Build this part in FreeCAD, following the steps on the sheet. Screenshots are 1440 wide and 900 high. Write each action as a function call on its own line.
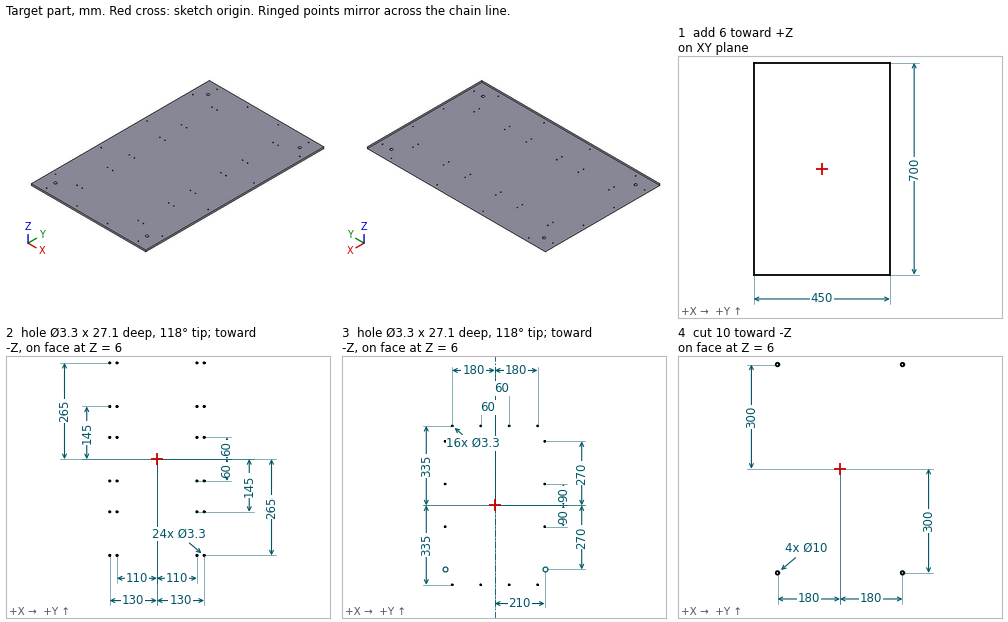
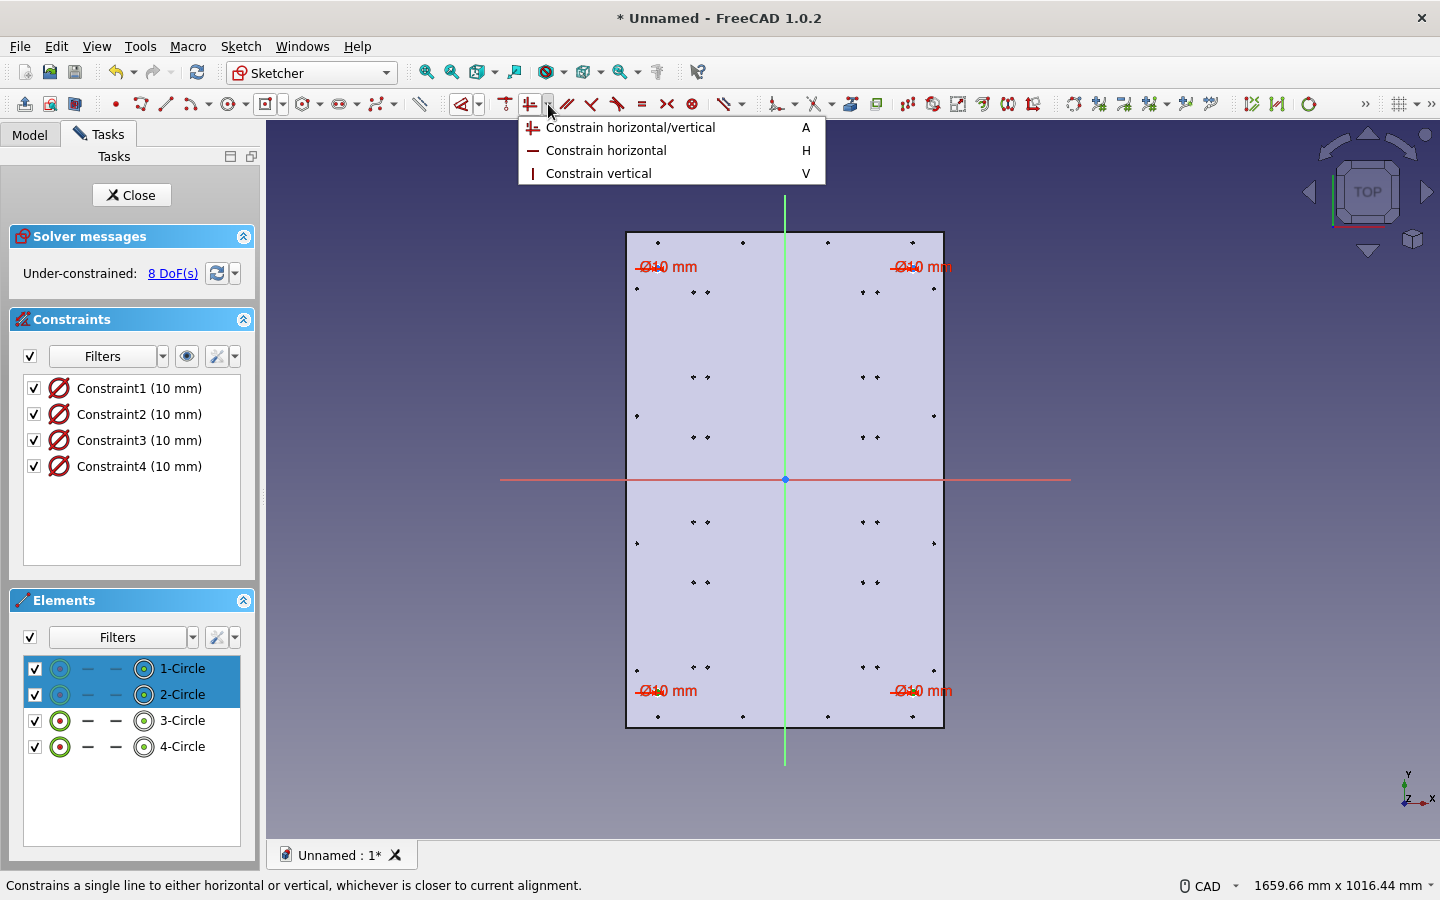
click(672, 150)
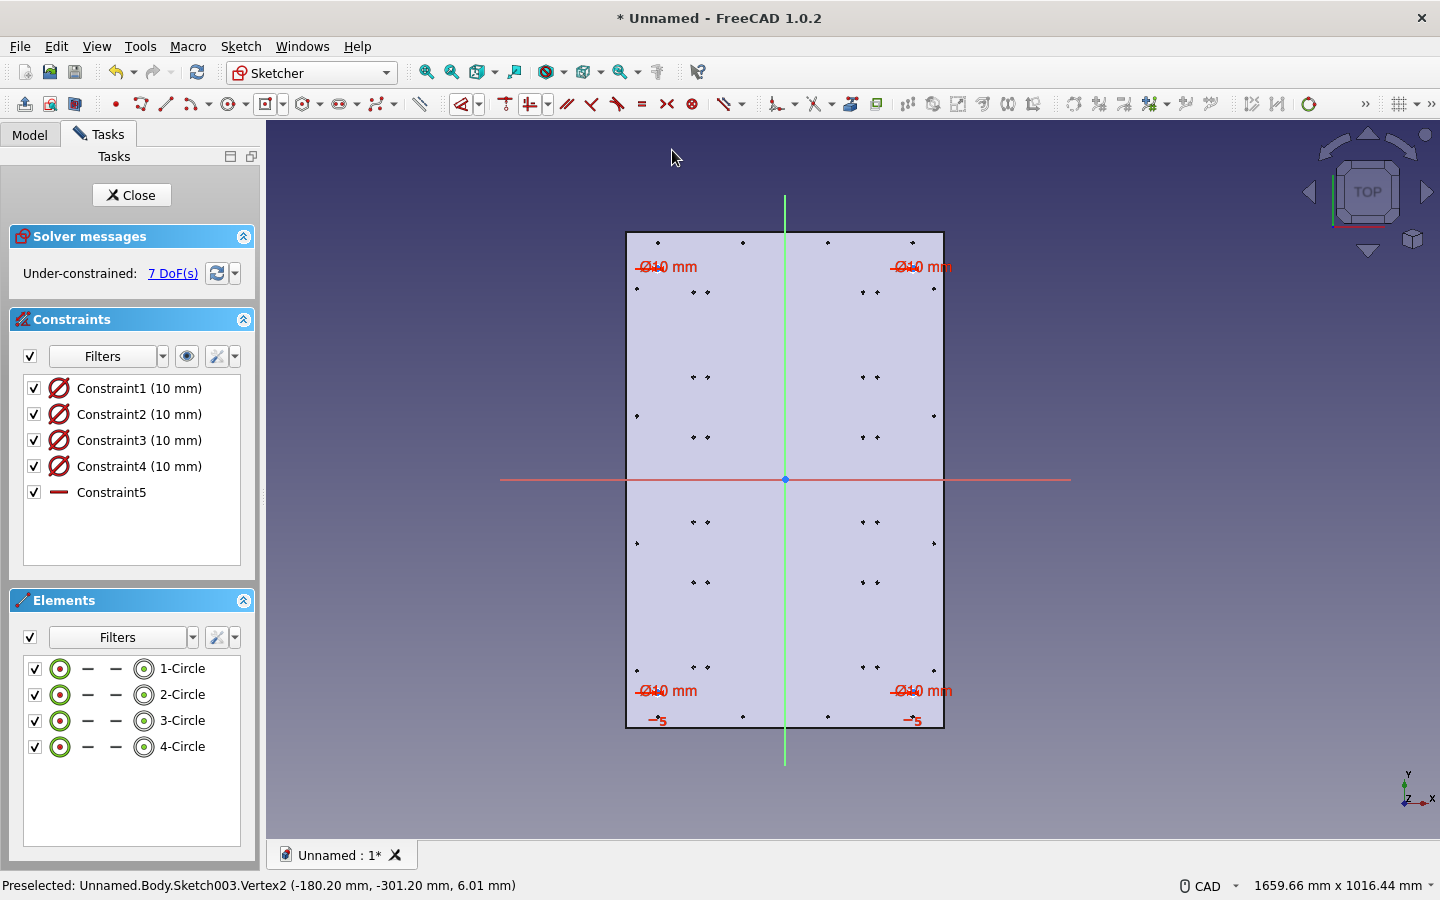
click(658, 693)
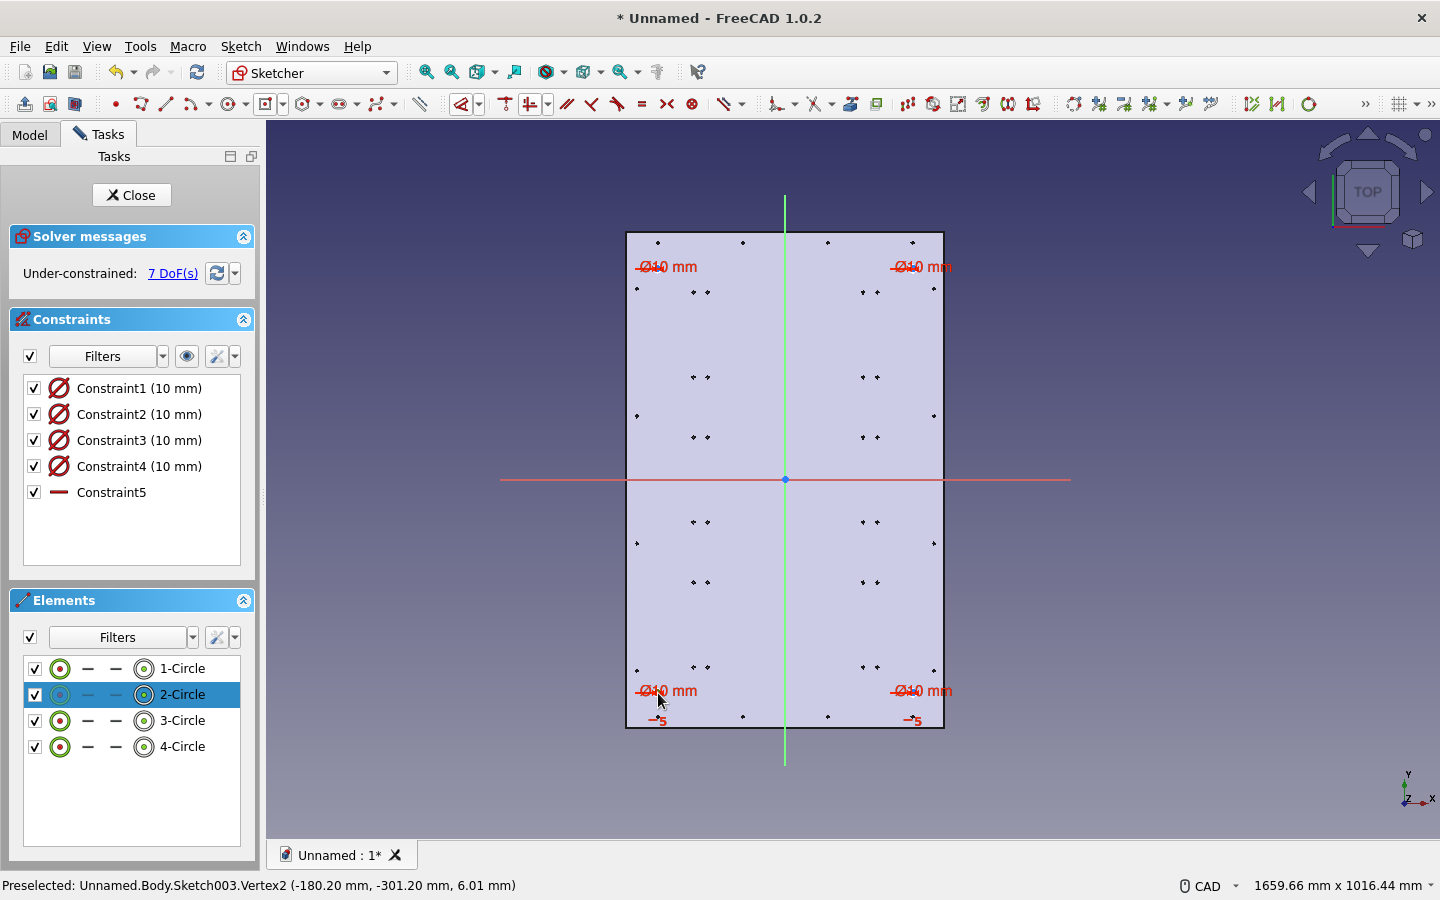
click(658, 269)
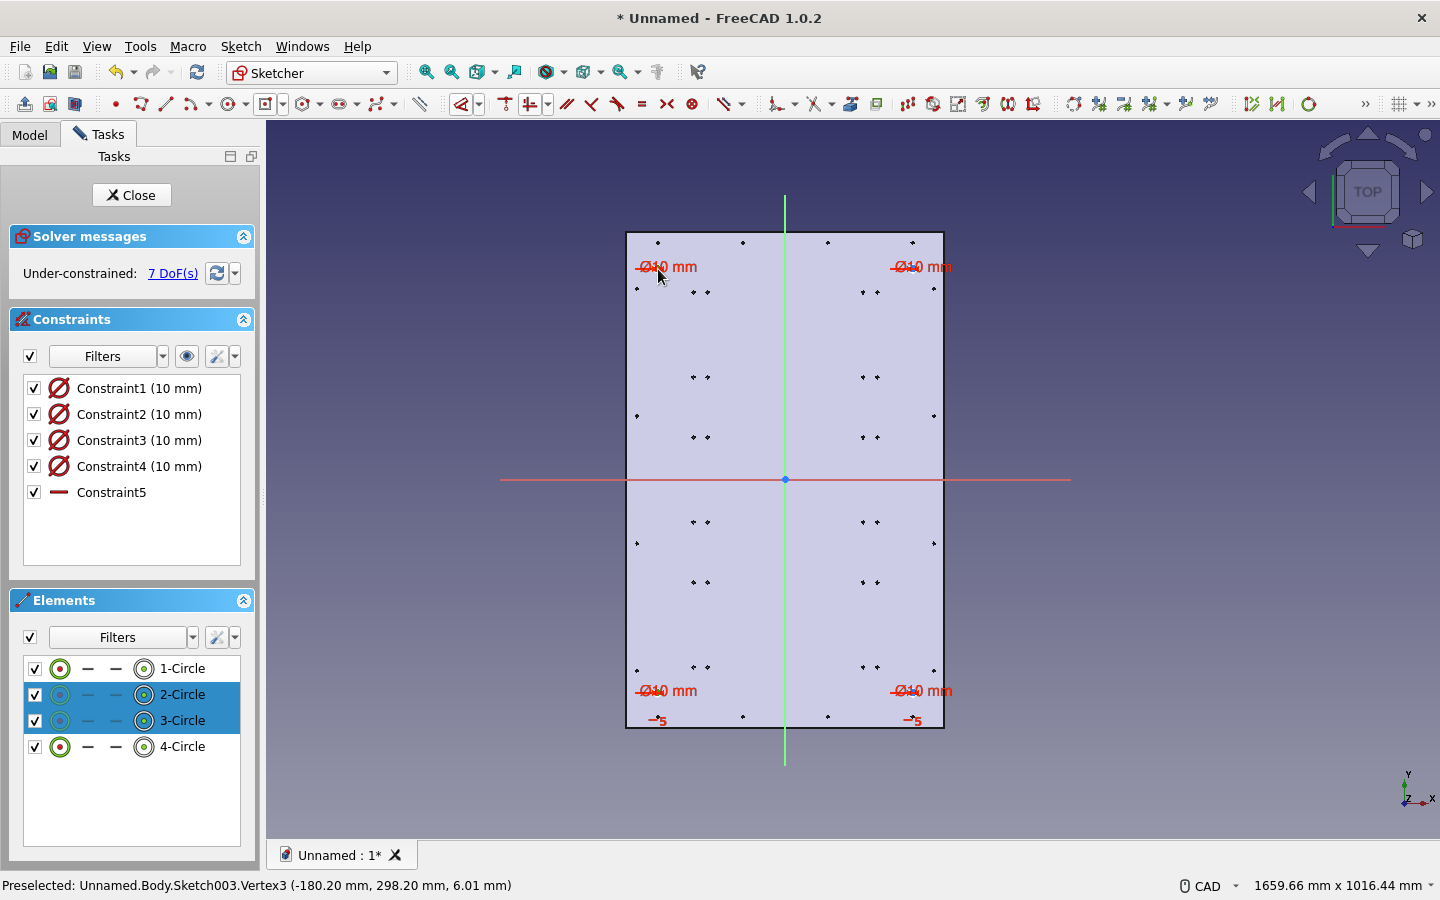
click(548, 104)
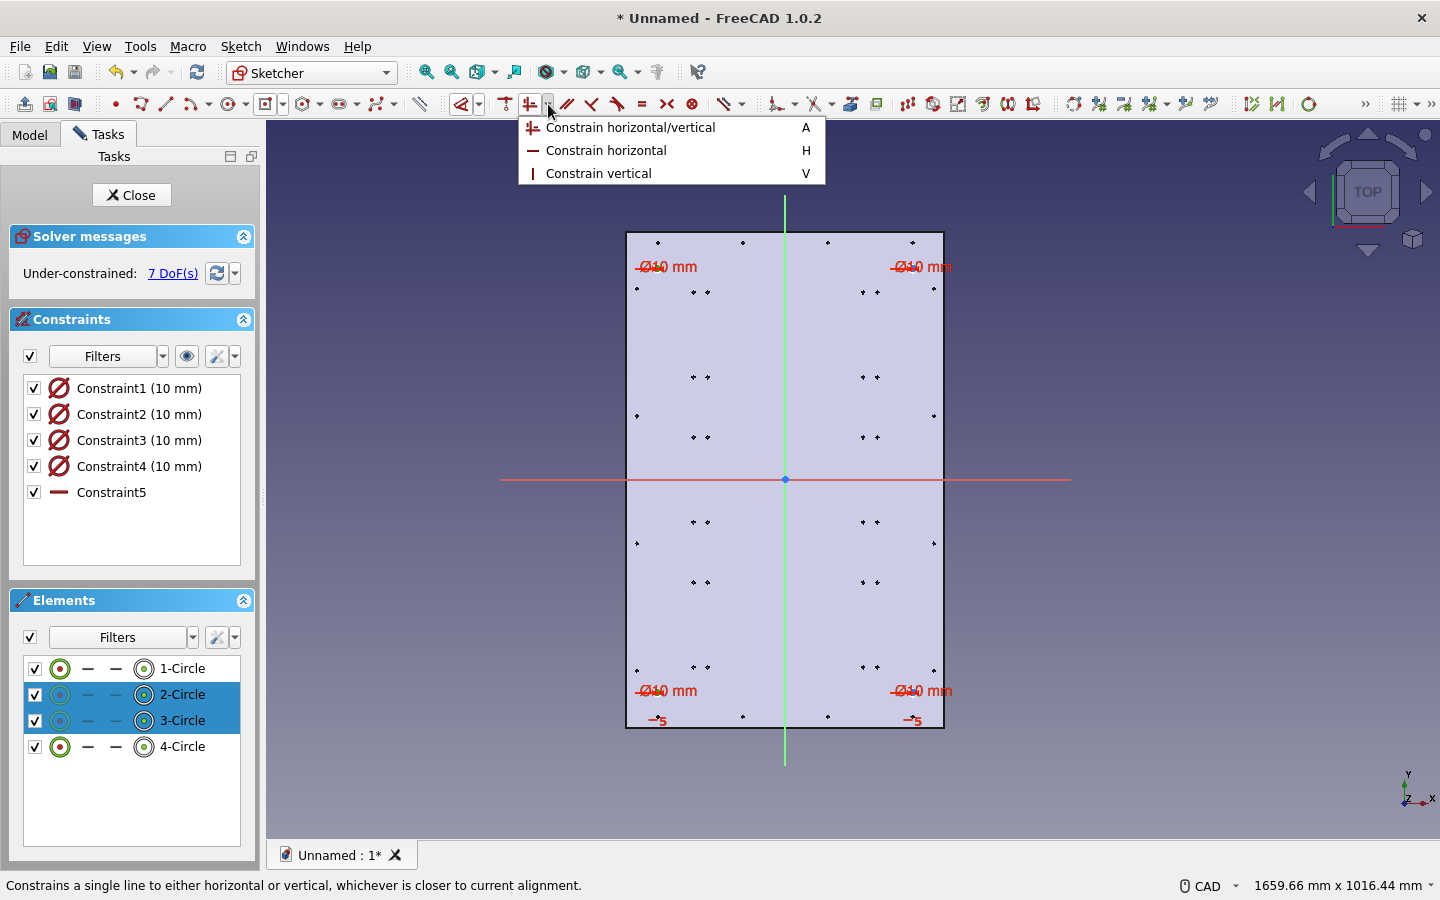
click(672, 174)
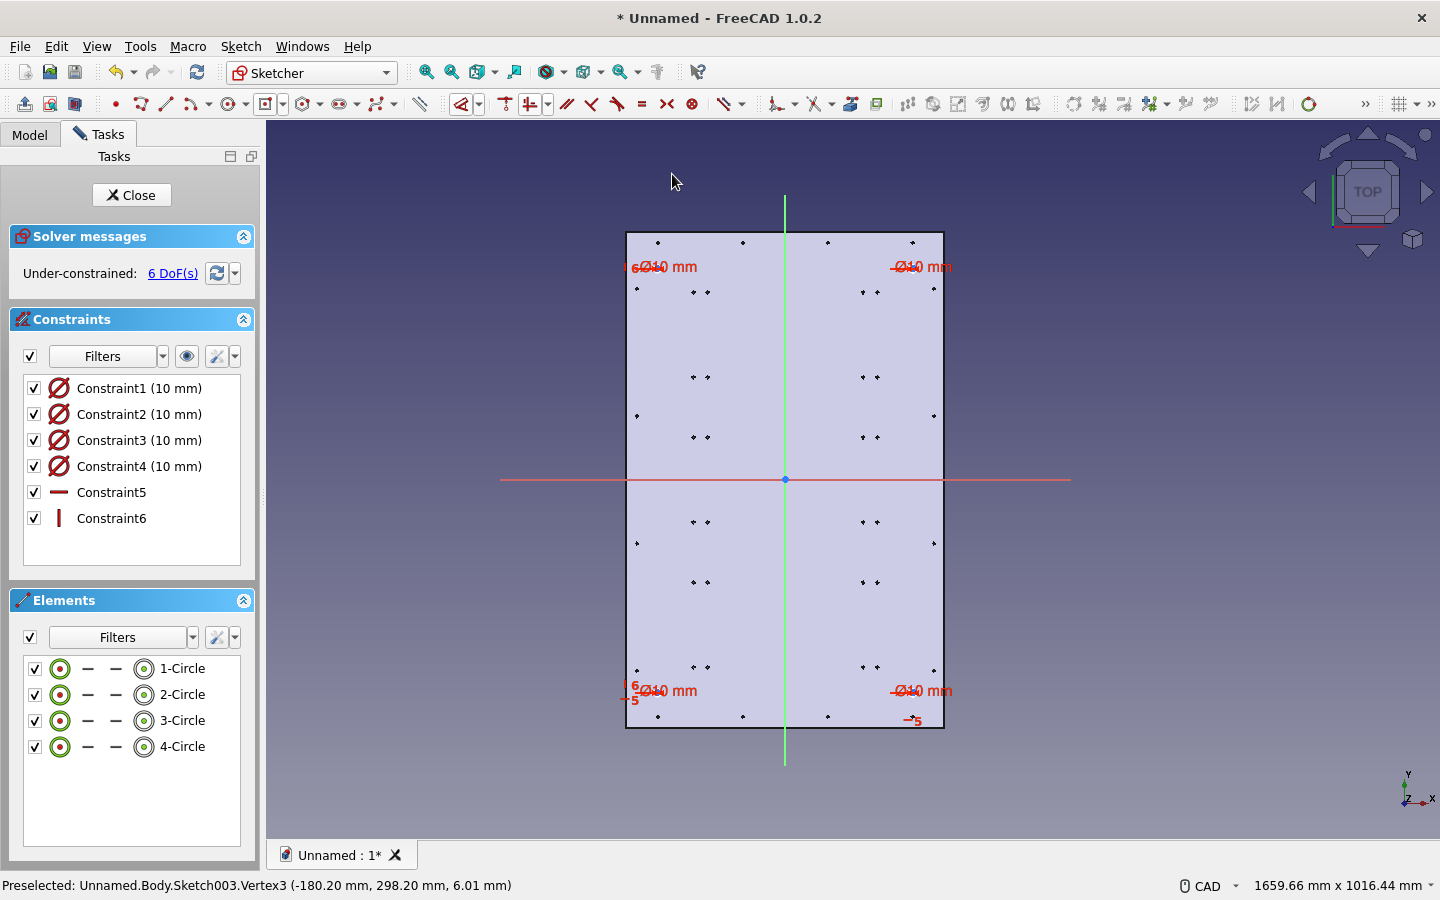
click(913, 693)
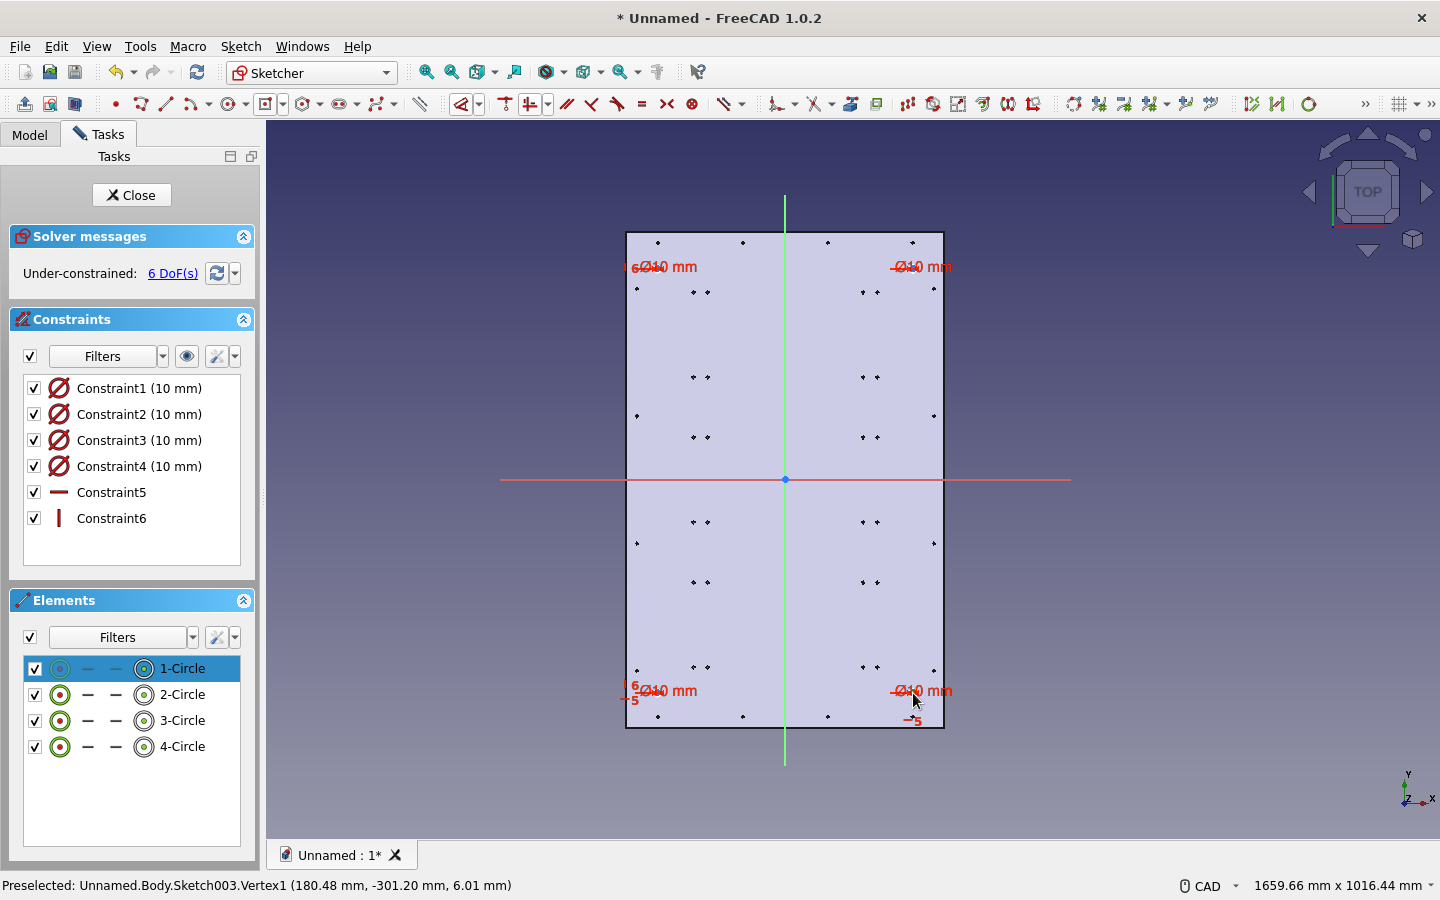
click(913, 269)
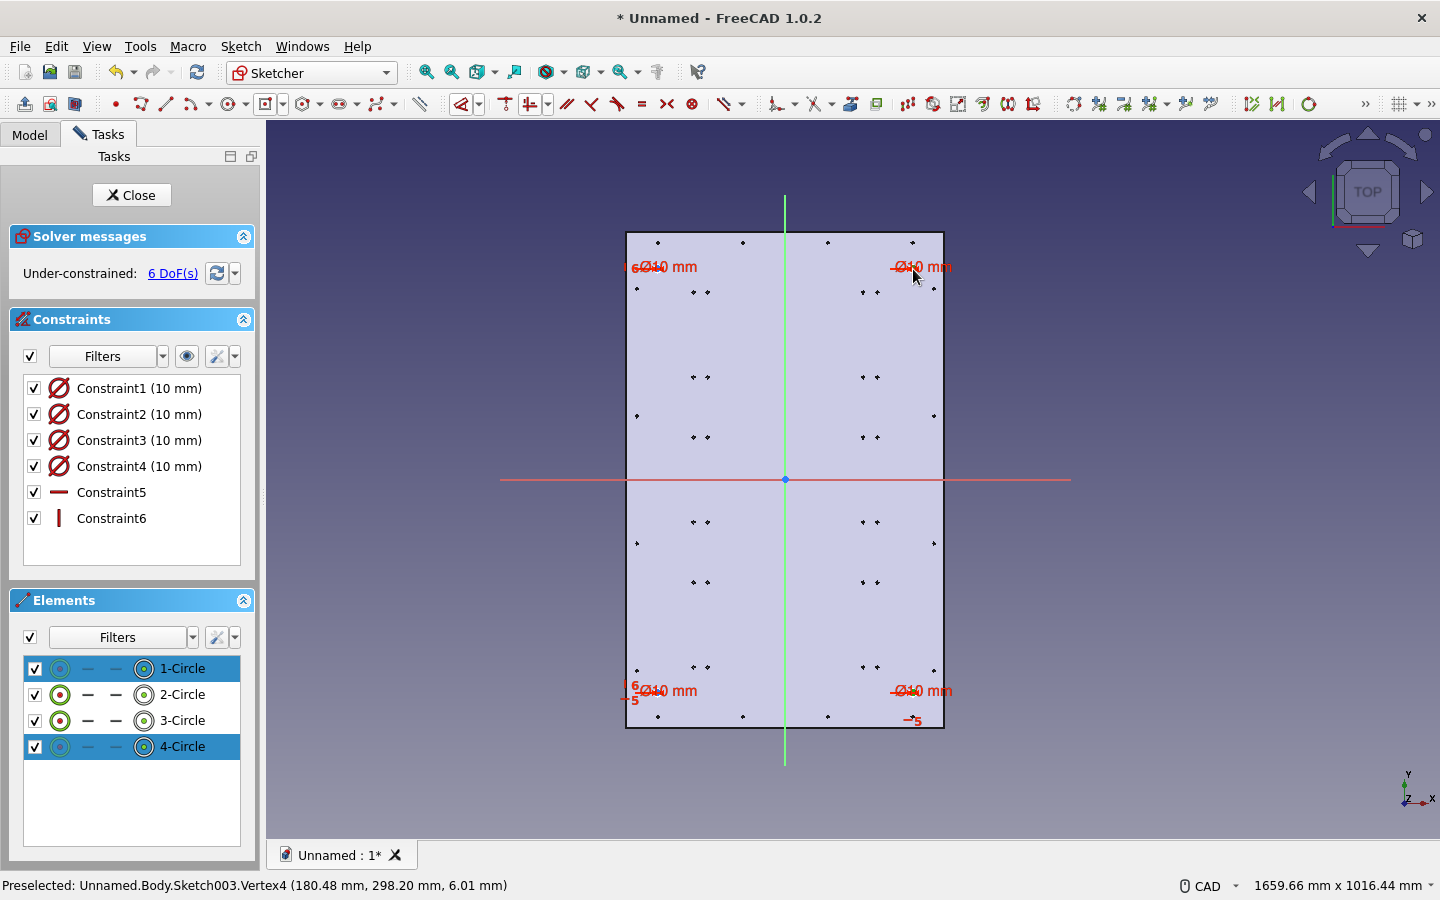
click(548, 104)